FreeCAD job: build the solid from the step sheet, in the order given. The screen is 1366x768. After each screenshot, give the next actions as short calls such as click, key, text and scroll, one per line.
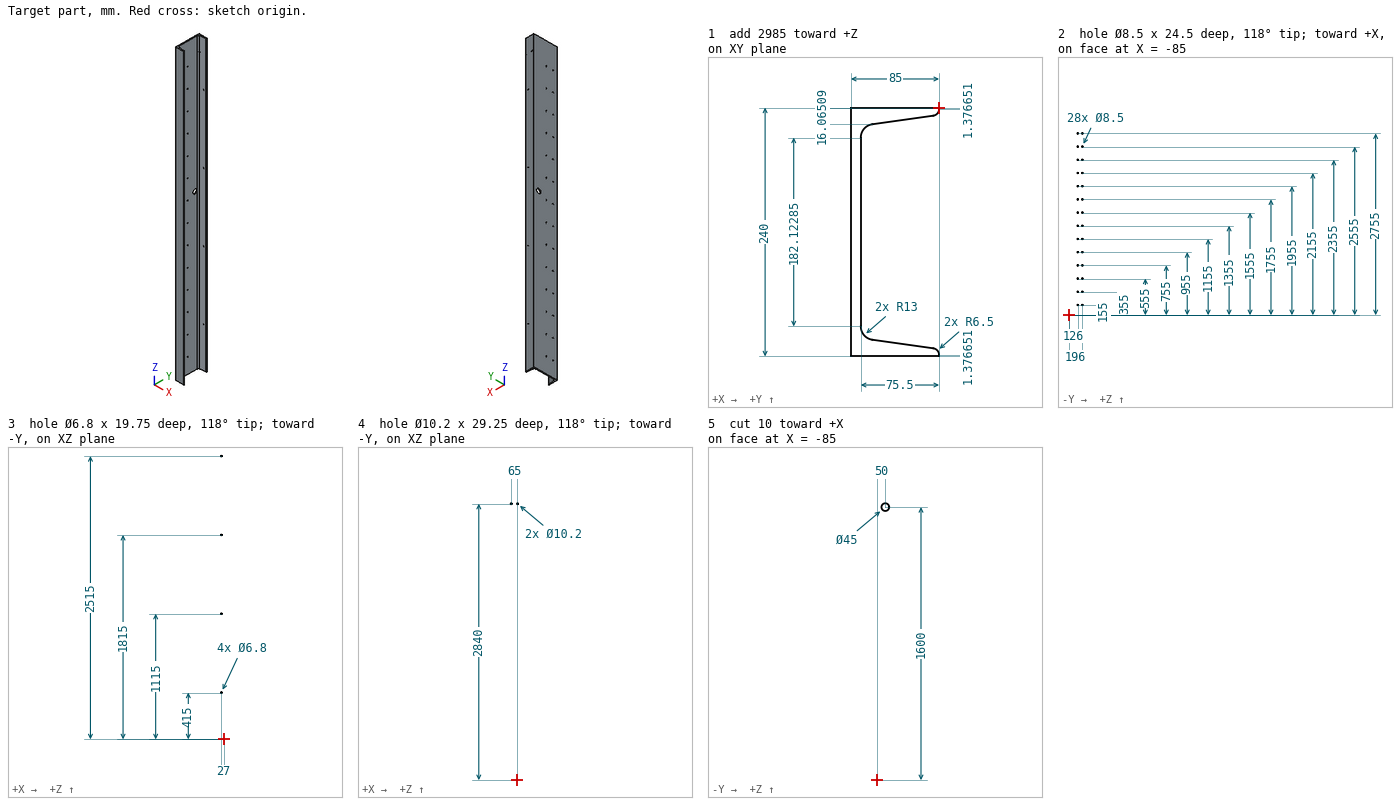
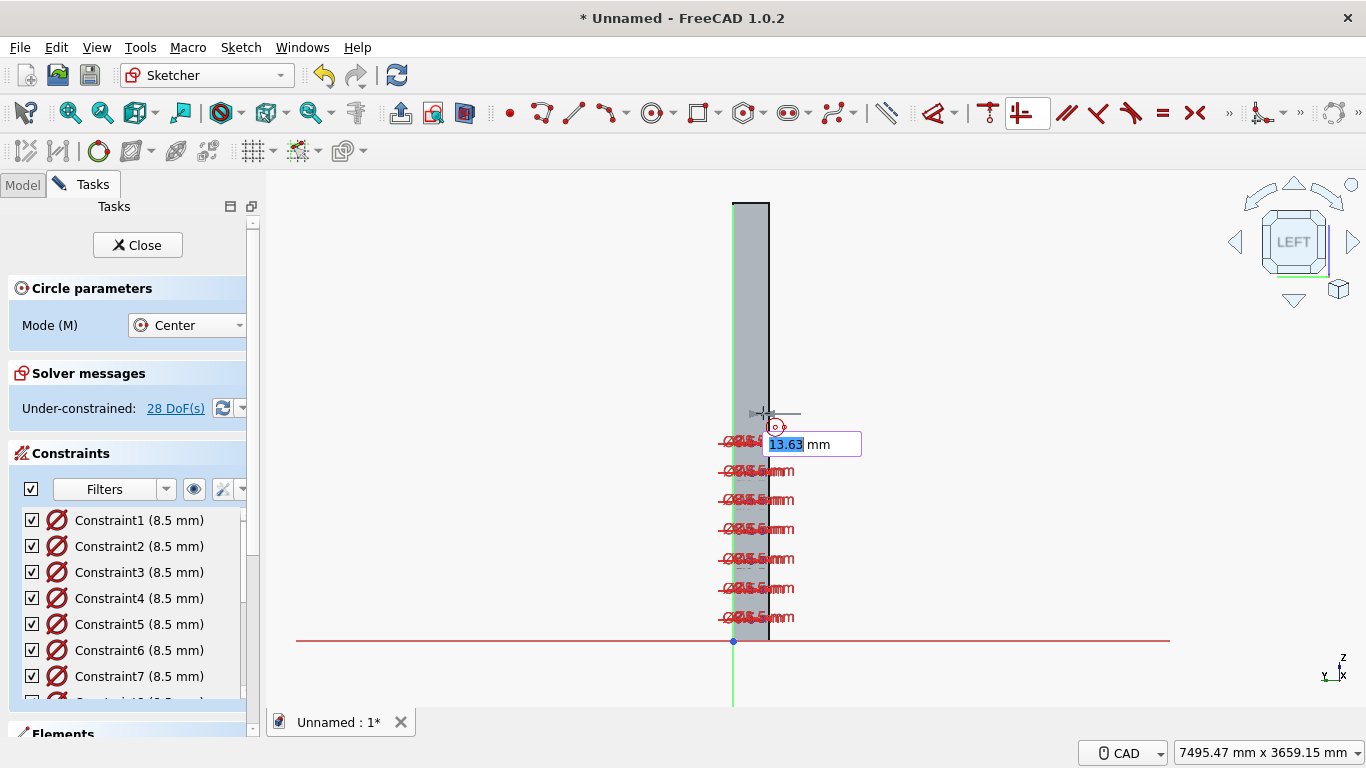
text(8.5)
key(Return)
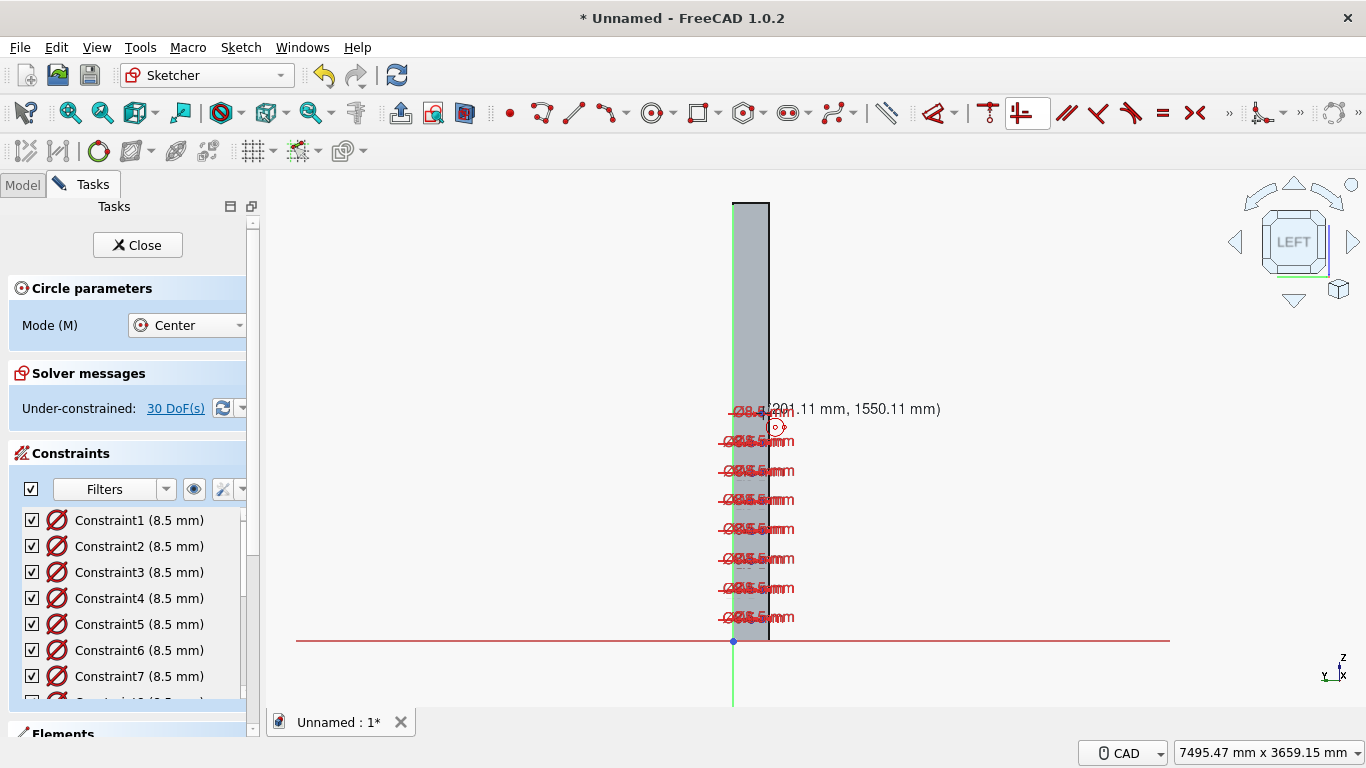
scroll(752, 413, up, 18)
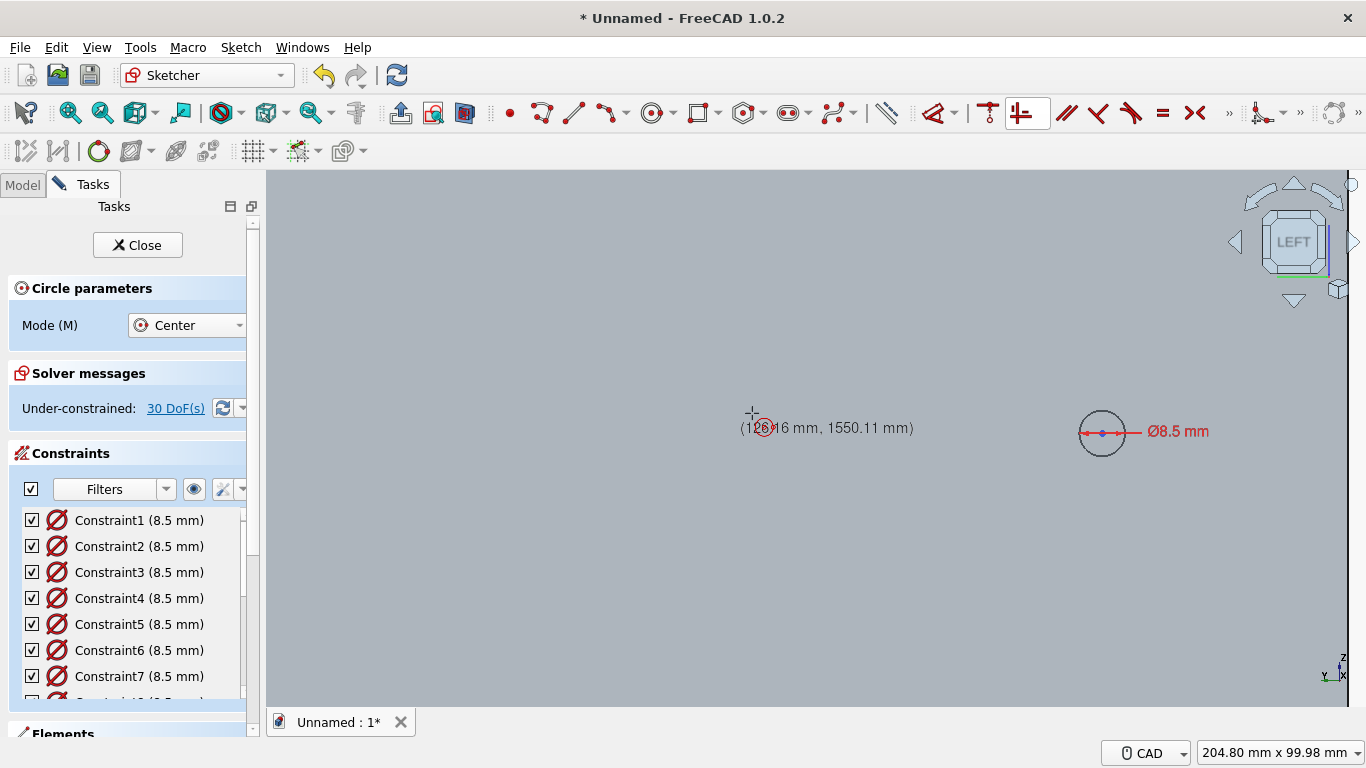
scroll(752, 413, down, 18)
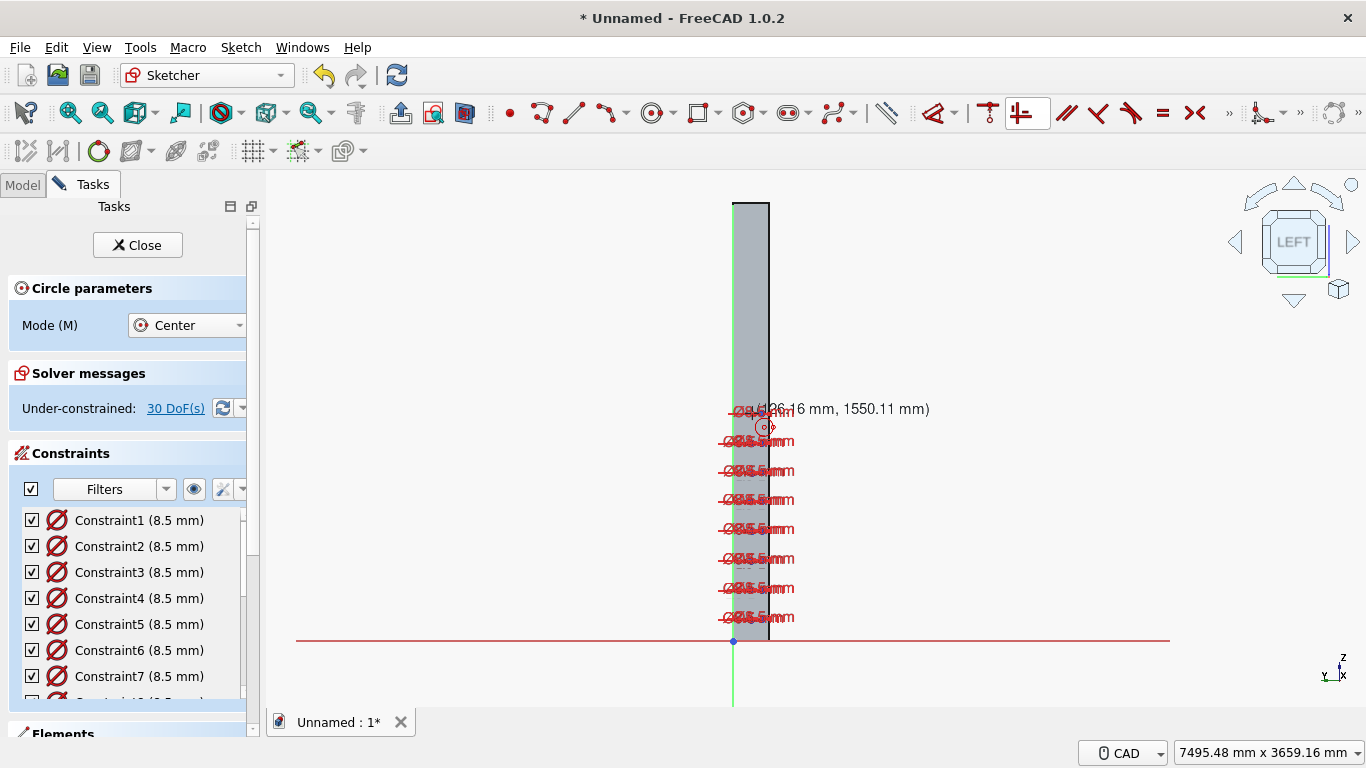
scroll(752, 413, up, 3)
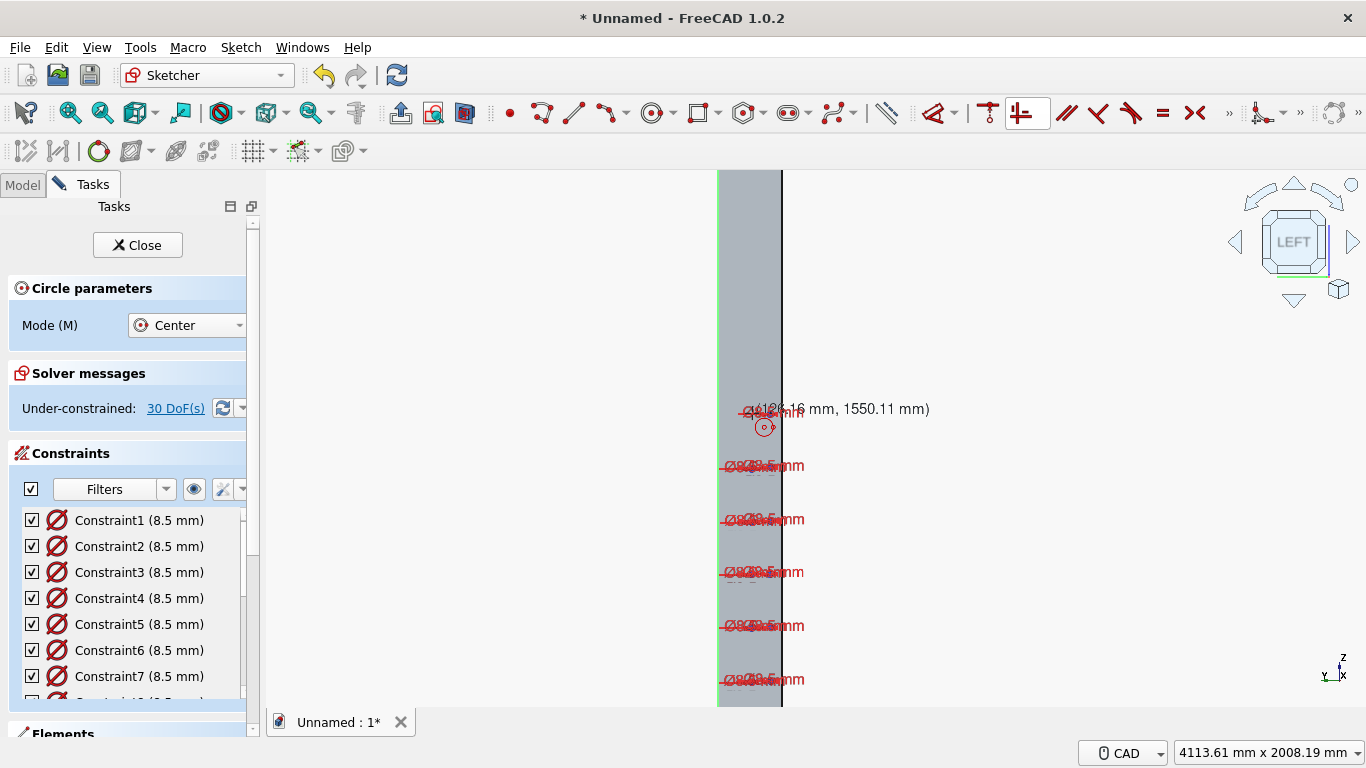
click(752, 413)
move(752, 412)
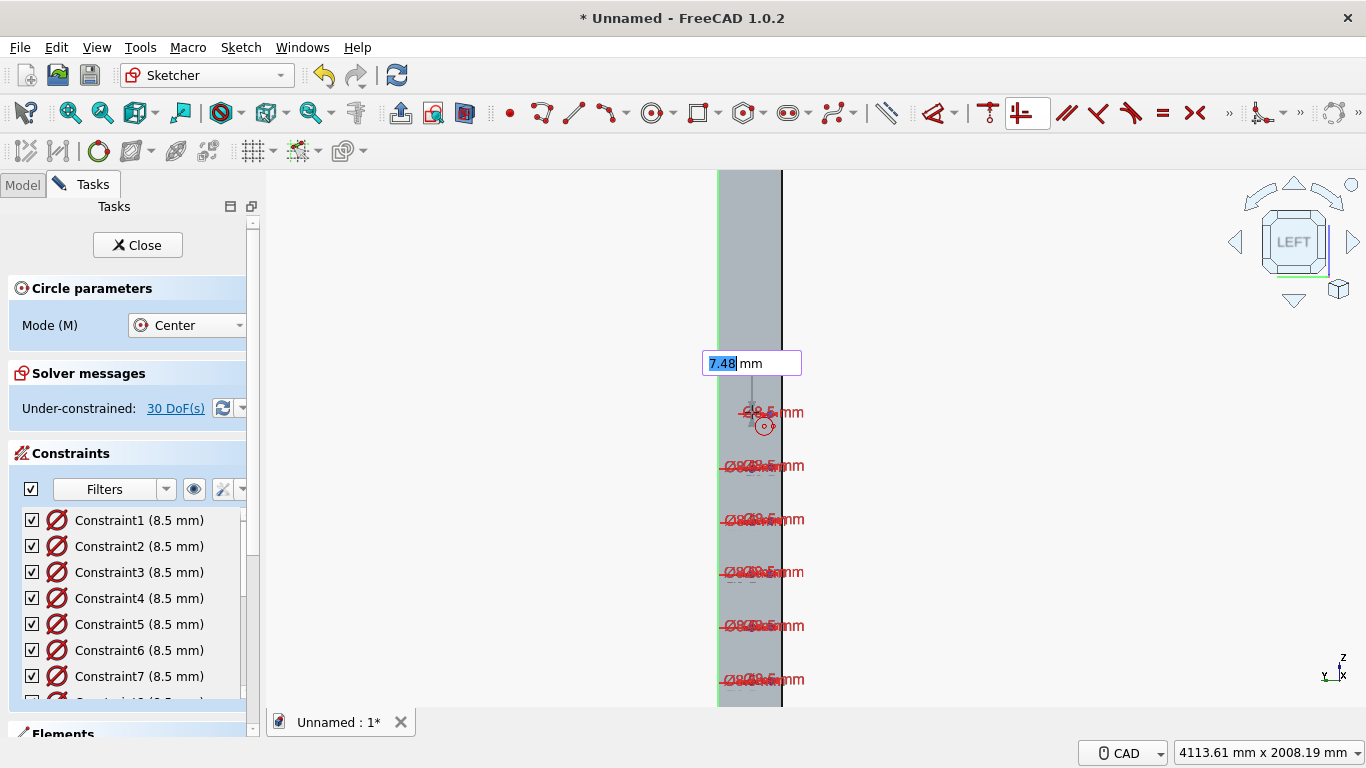
text(8.5)
key(Return)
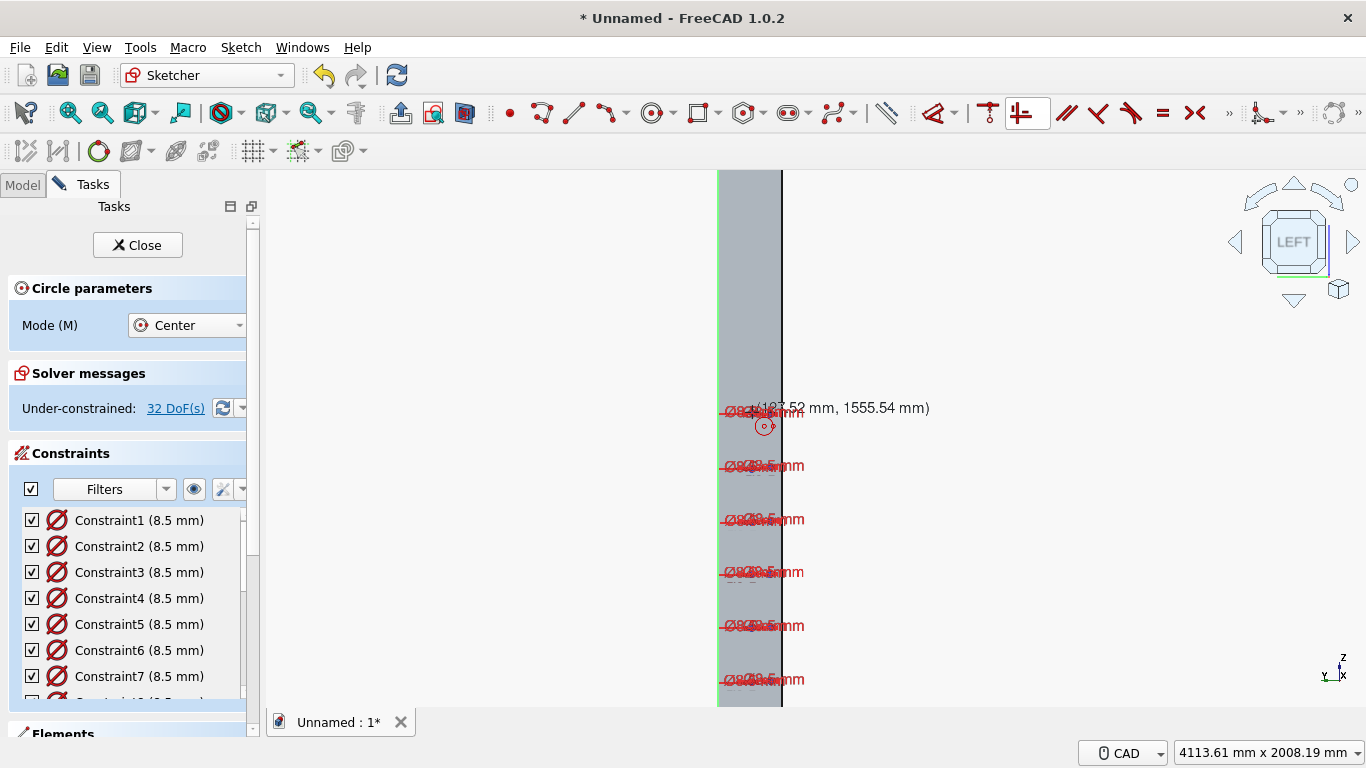
scroll(770, 360, up, 15)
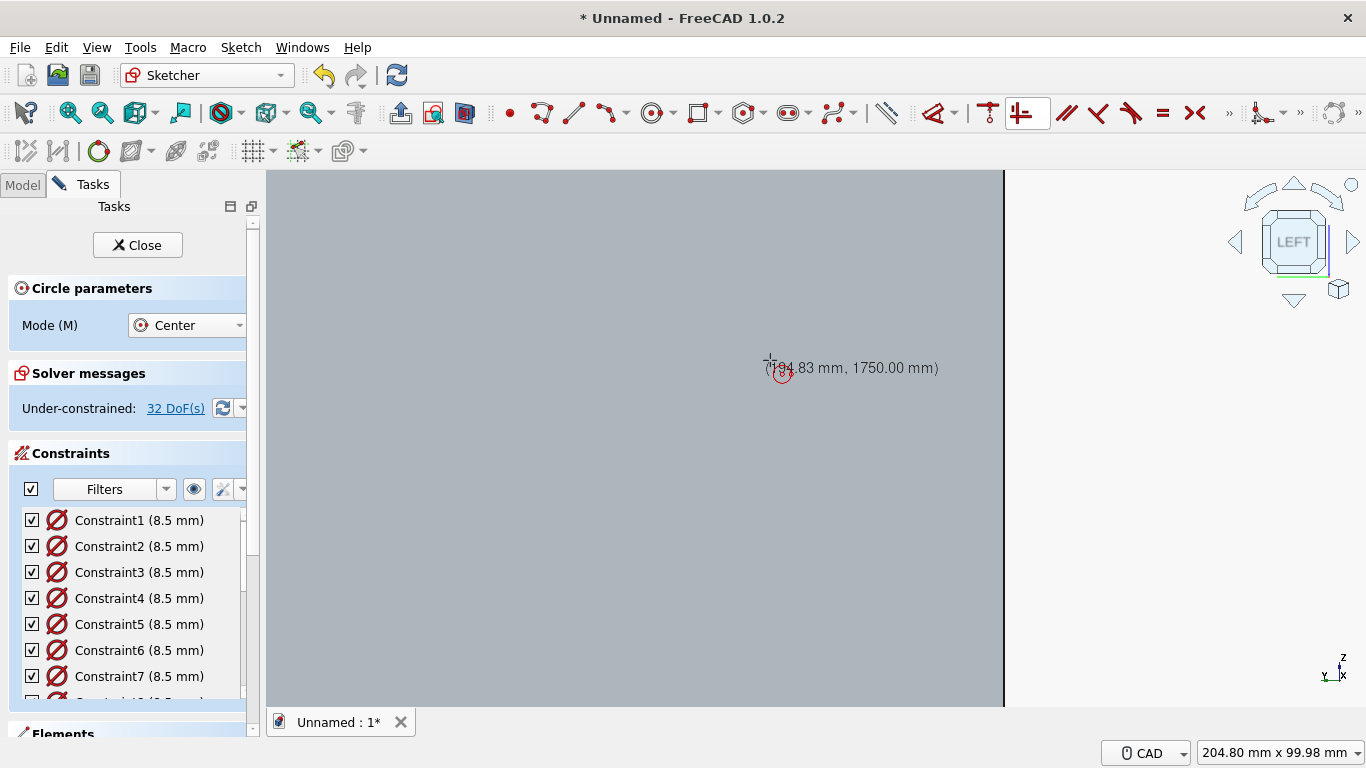
scroll(761, 384, down, 18)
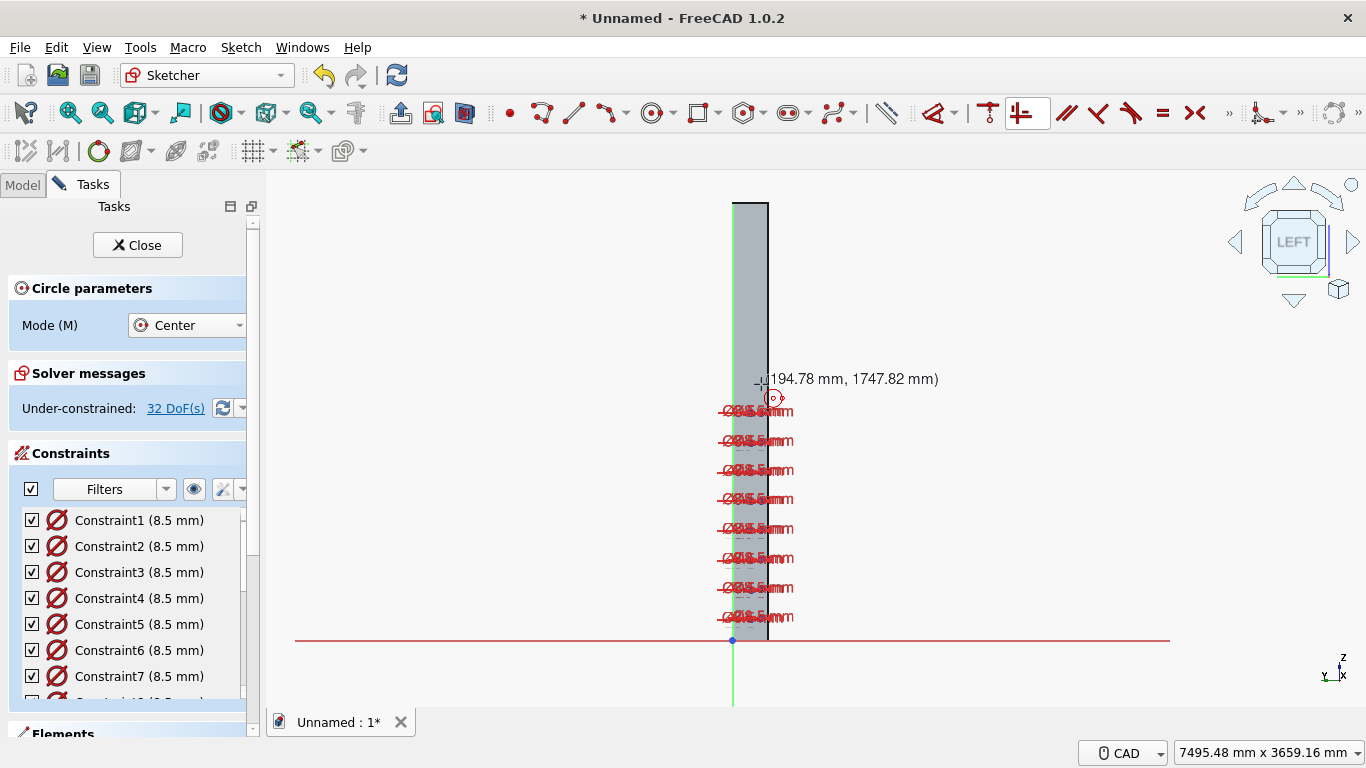
click(762, 383)
move(762, 383)